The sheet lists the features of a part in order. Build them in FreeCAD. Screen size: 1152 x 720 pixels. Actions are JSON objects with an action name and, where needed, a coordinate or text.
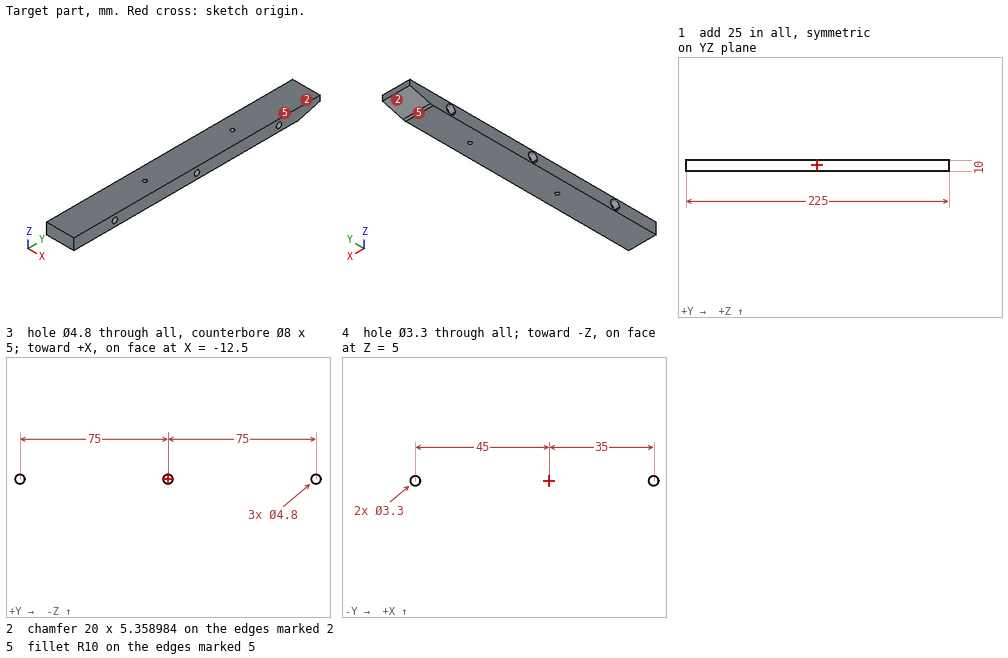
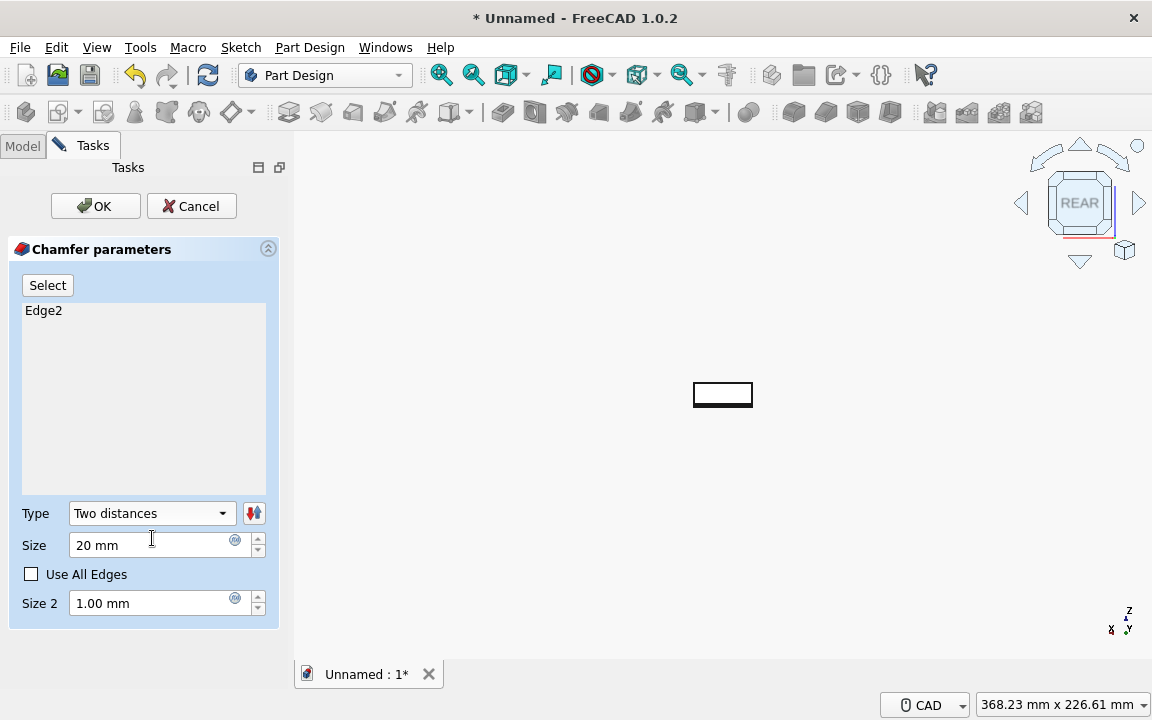
{"action": "triple_click", "coordinate": [160, 603]}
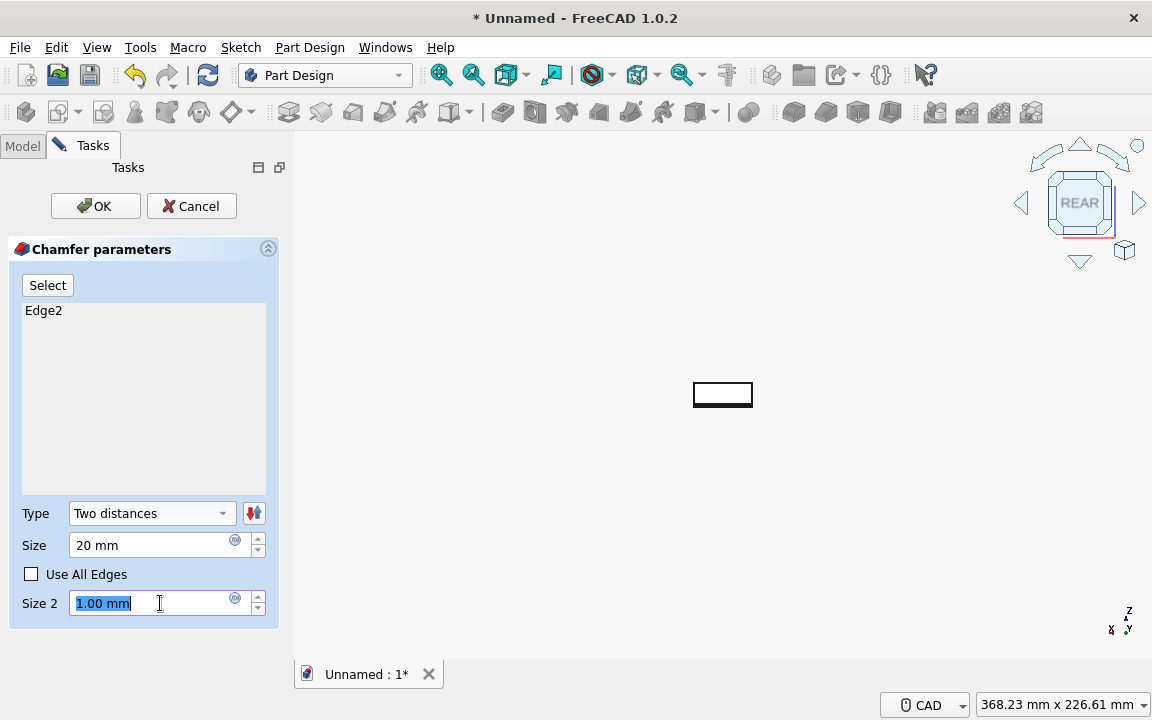
{"action": "type", "text": "5.358984"}
{"action": "key", "text": "Tab"}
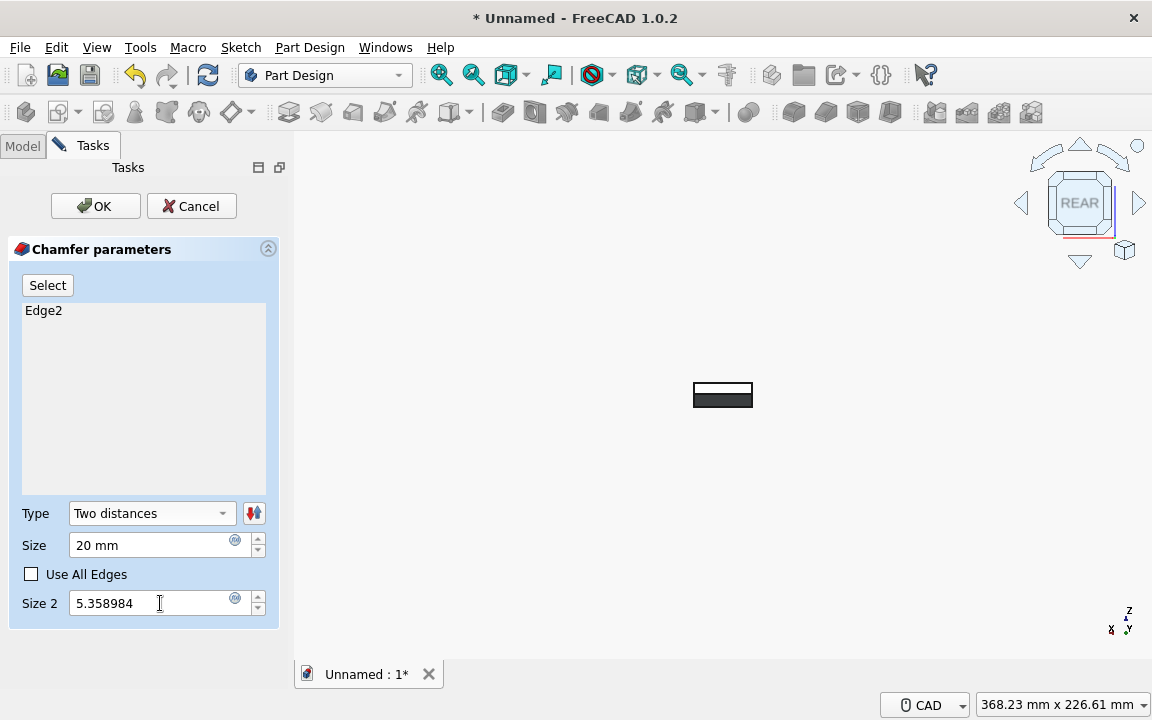
{"action": "left_click", "coordinate": [96, 206]}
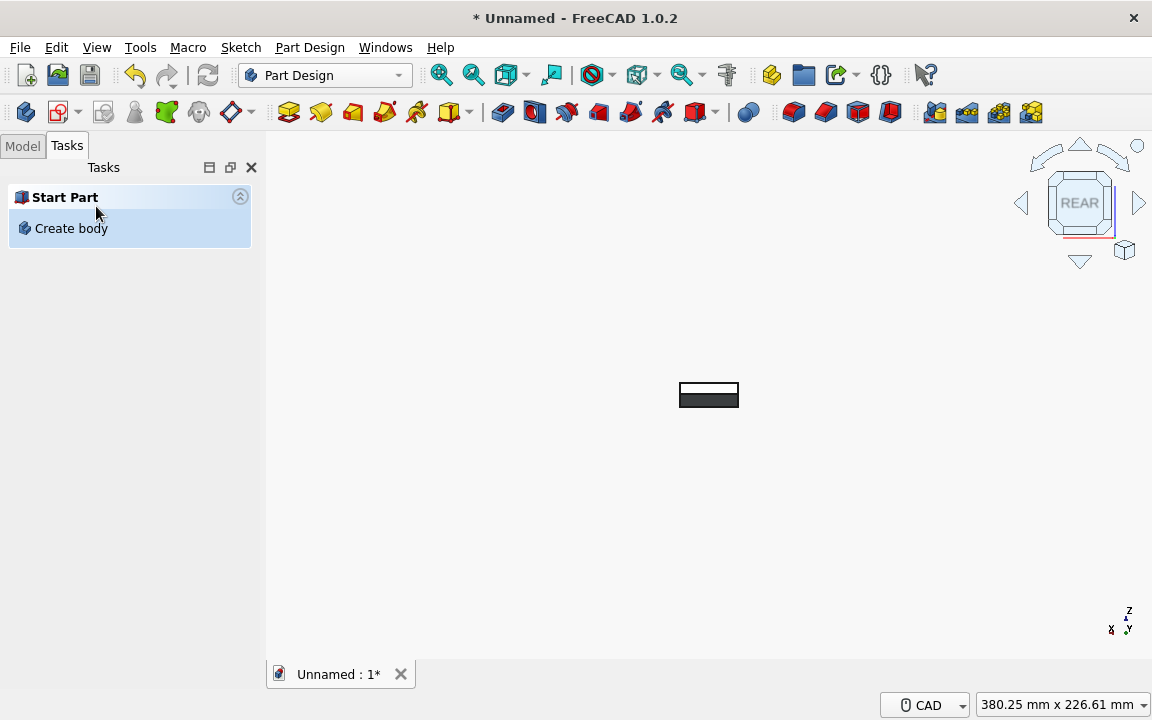
{"action": "left_click", "coordinate": [442, 76]}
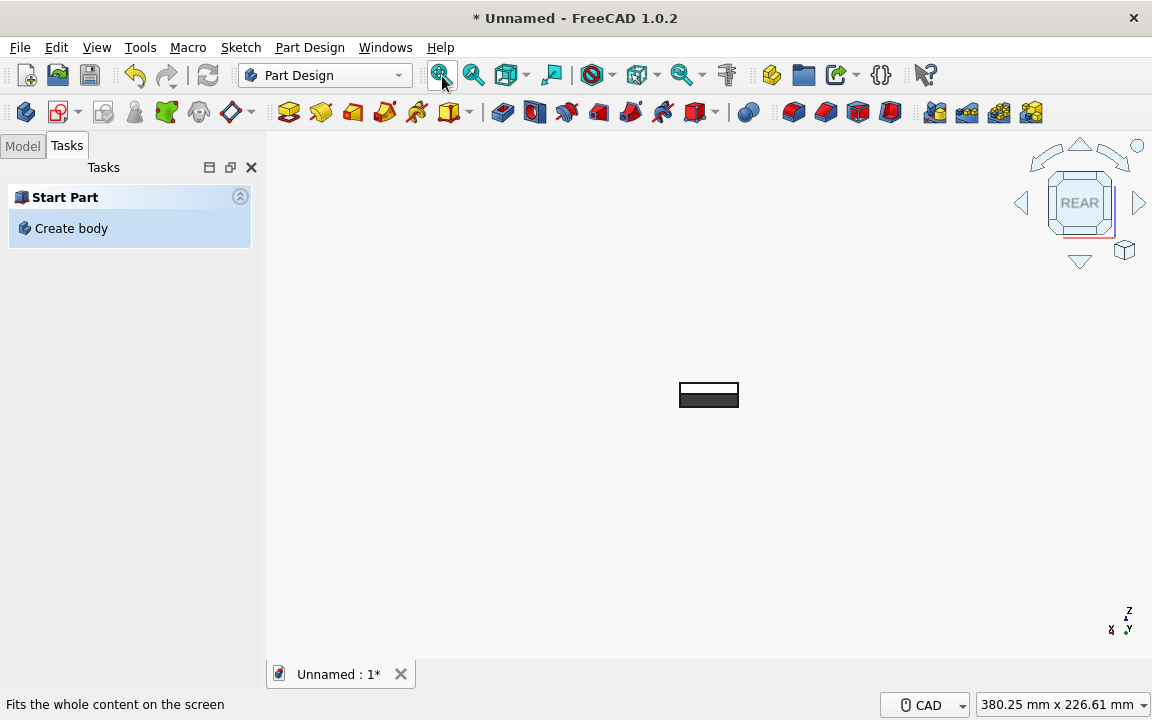
{"action": "key", "text": "6"}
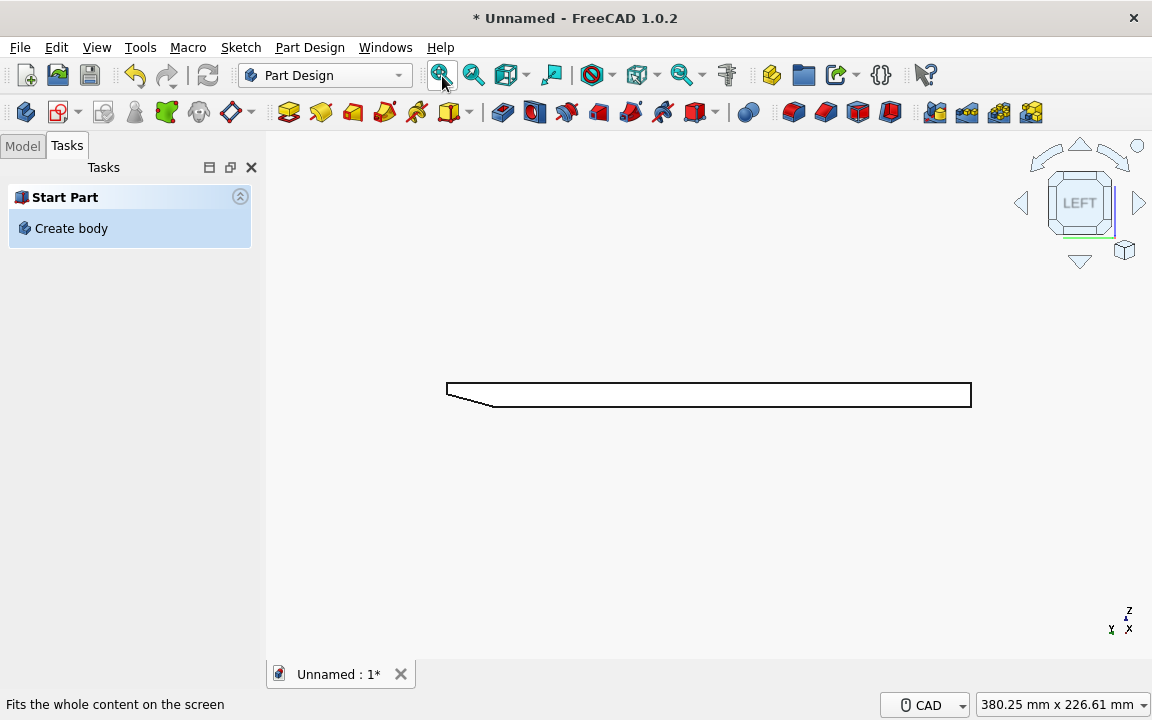
{"action": "left_click", "coordinate": [859, 394]}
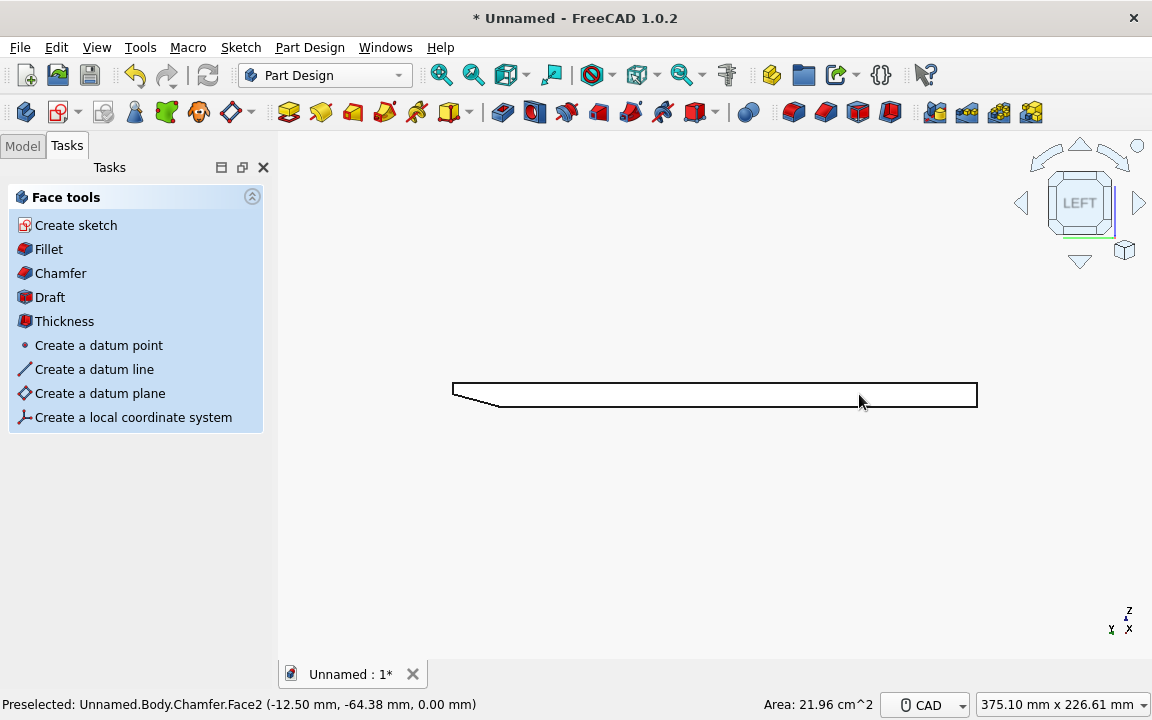
{"action": "left_click", "coordinate": [58, 112]}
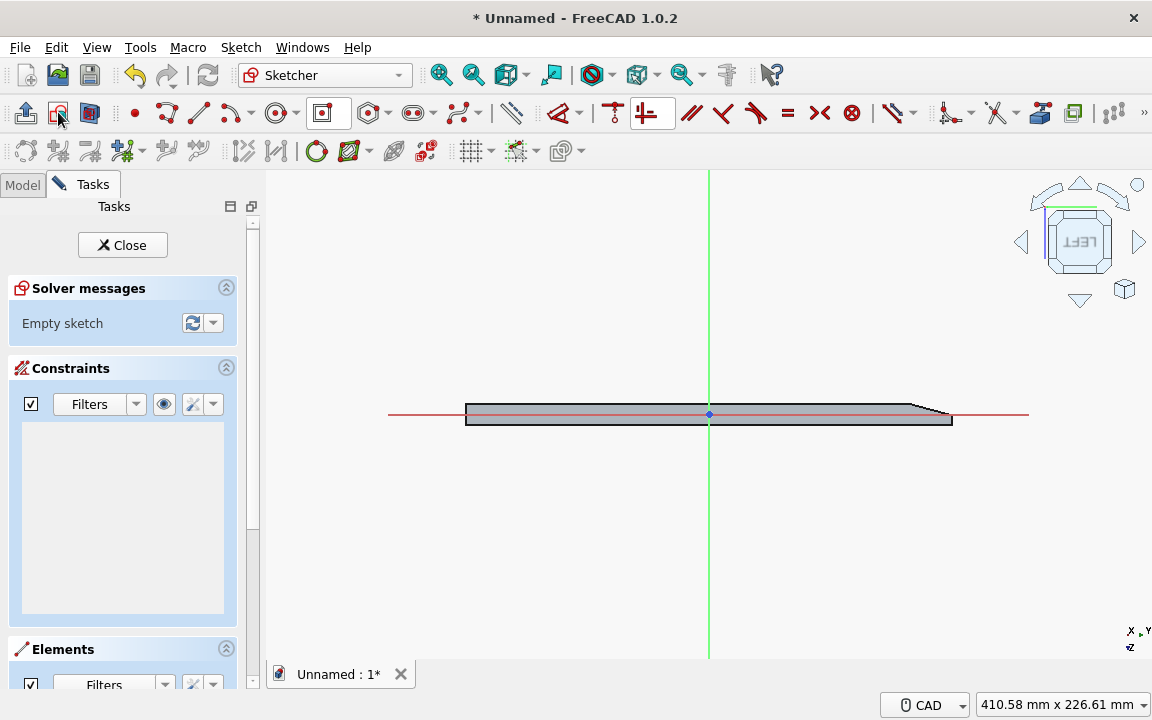
{"action": "scroll", "coordinate": [848, 414], "scroll_direction": "up", "scroll_amount": 2}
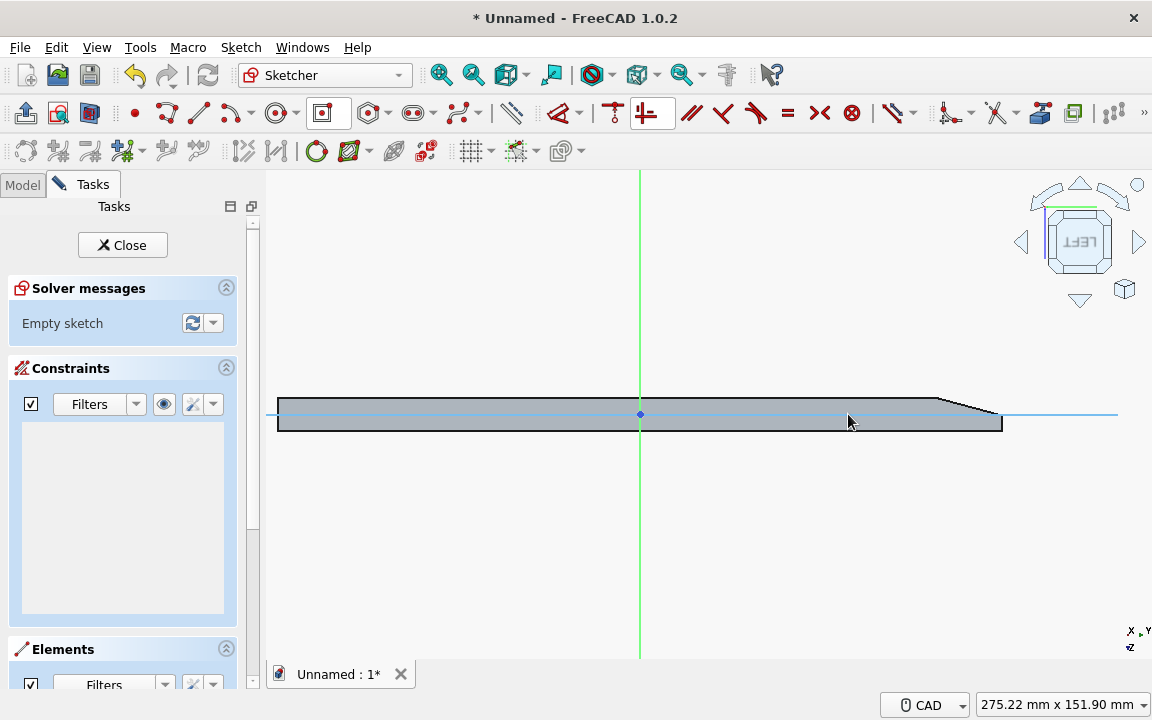
{"action": "left_click", "coordinate": [276, 114]}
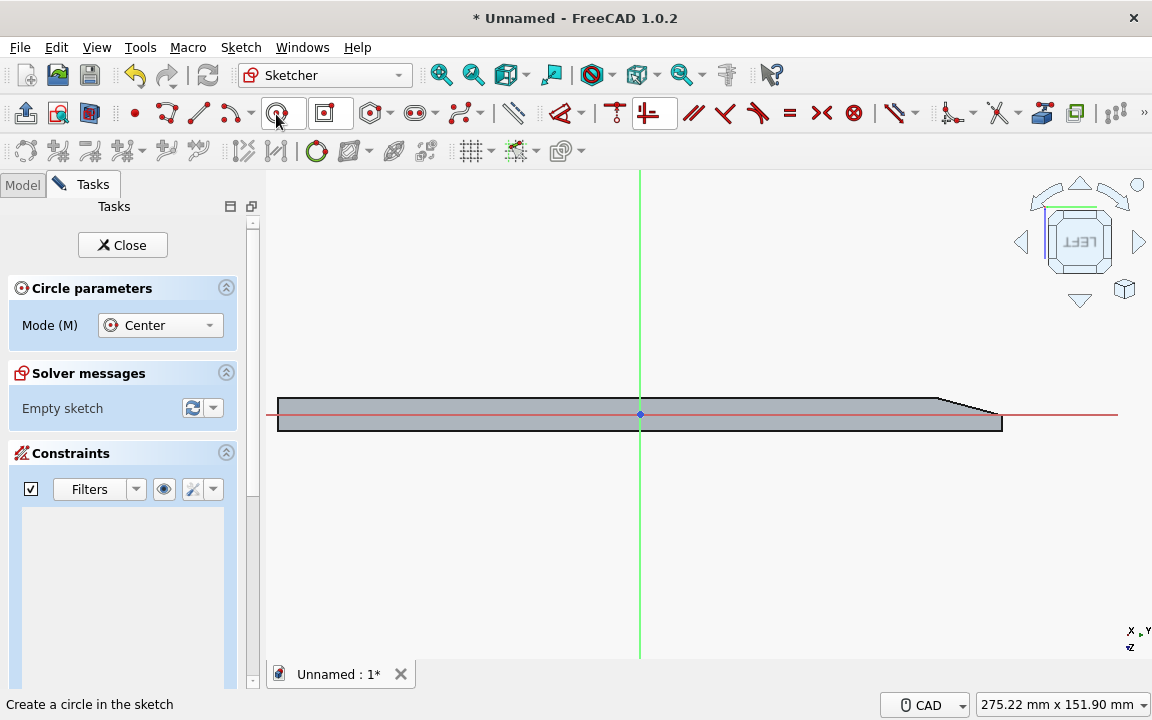
{"action": "scroll", "coordinate": [882, 414], "scroll_direction": "up", "scroll_amount": 6}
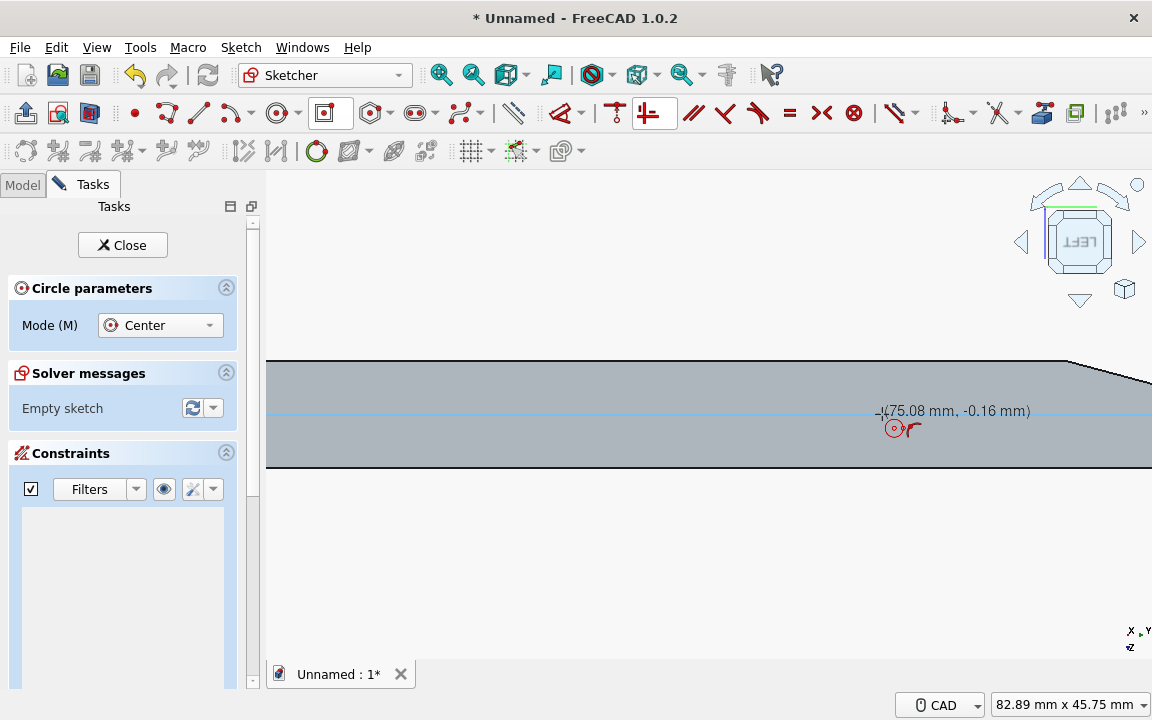
{"action": "left_click", "coordinate": [880, 414]}
{"action": "left_click", "coordinate": [898, 396]}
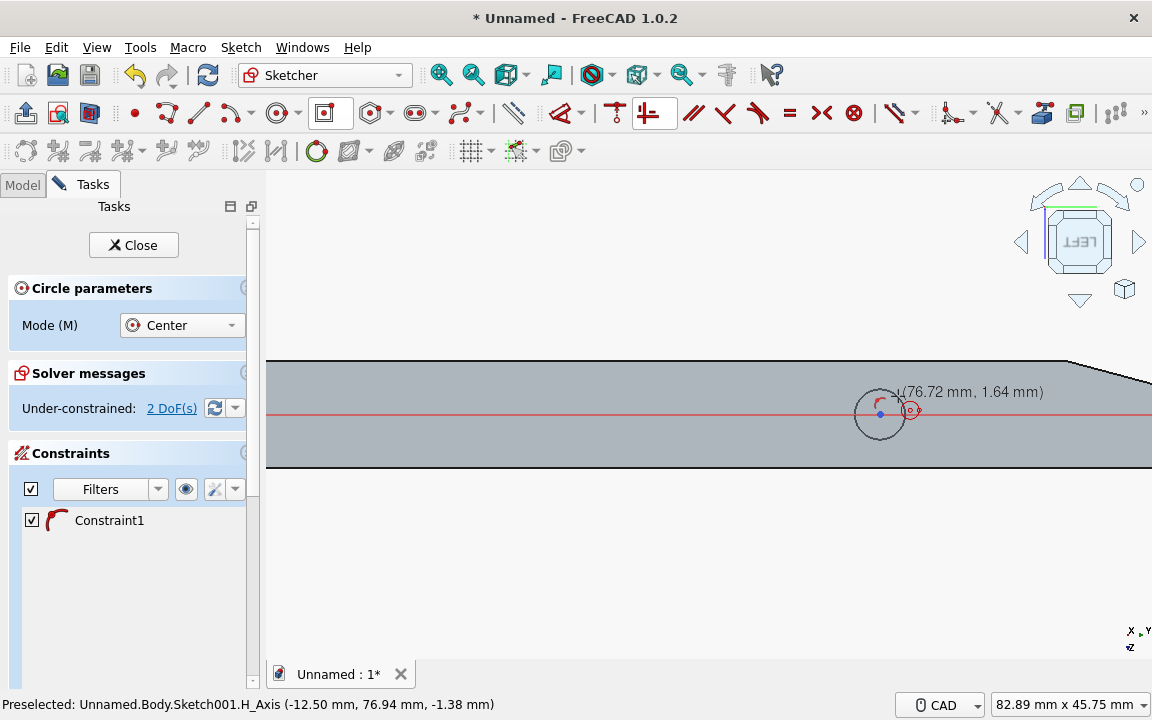
{"action": "scroll", "coordinate": [883, 414], "scroll_direction": "down", "scroll_amount": 6}